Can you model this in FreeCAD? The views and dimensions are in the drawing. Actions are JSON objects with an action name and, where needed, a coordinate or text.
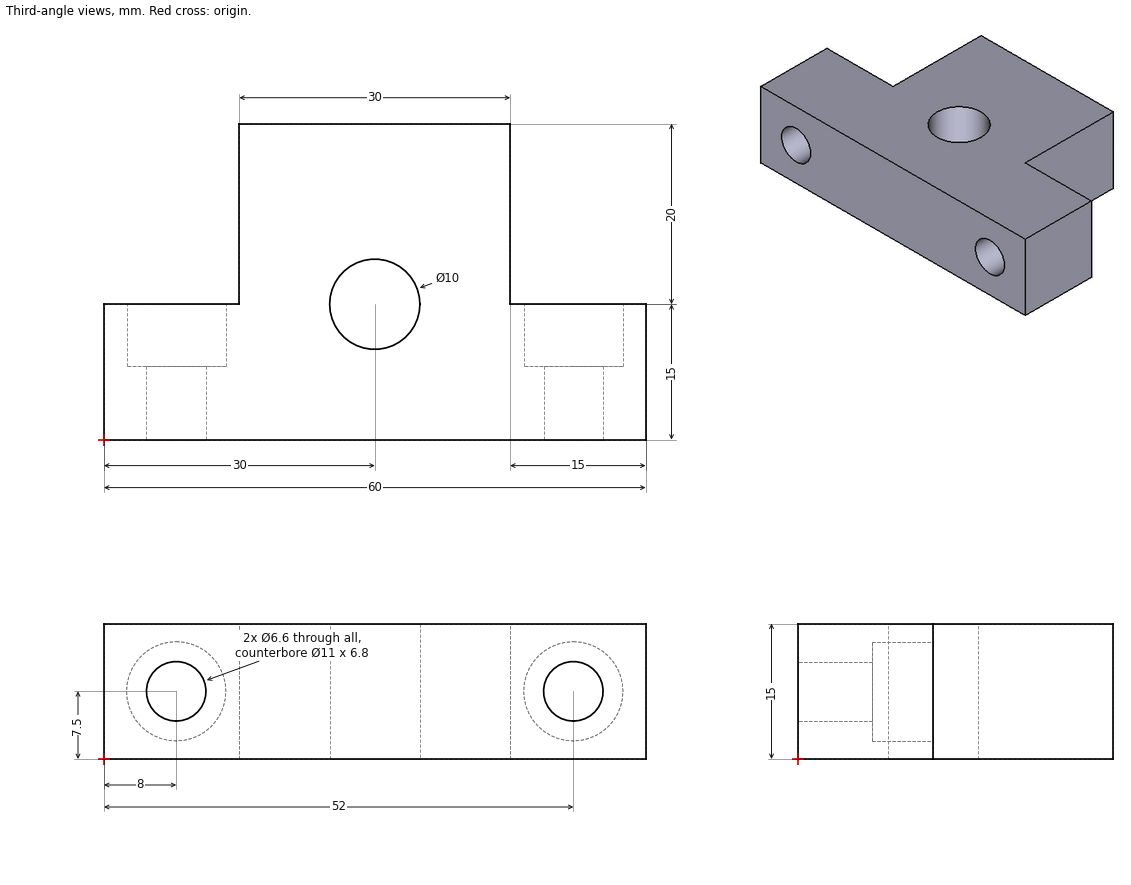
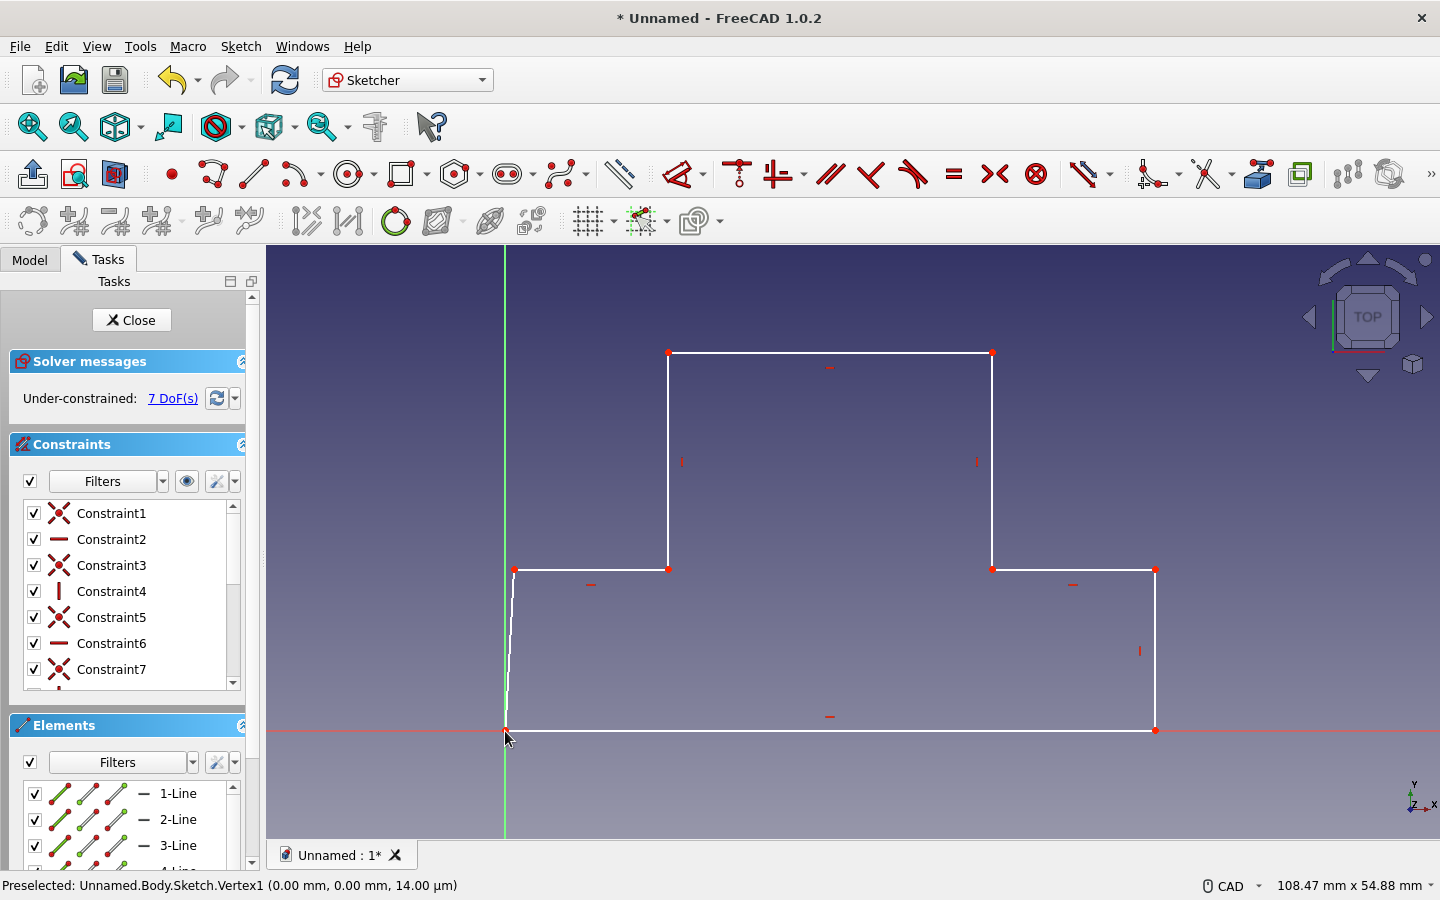
{"action": "left_click", "coordinate": [508, 683]}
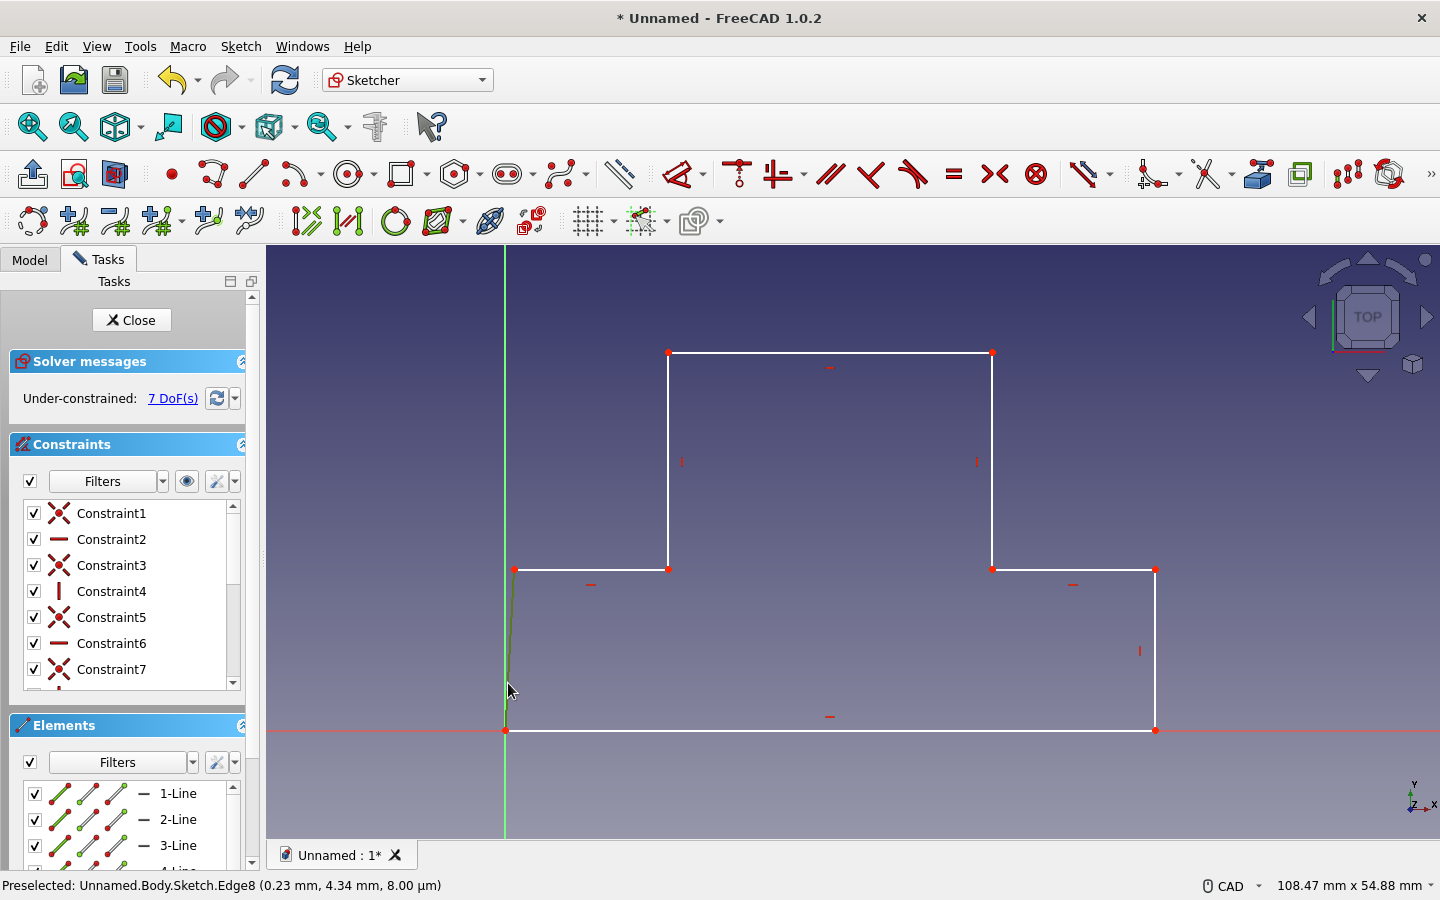
{"action": "key", "text": "v"}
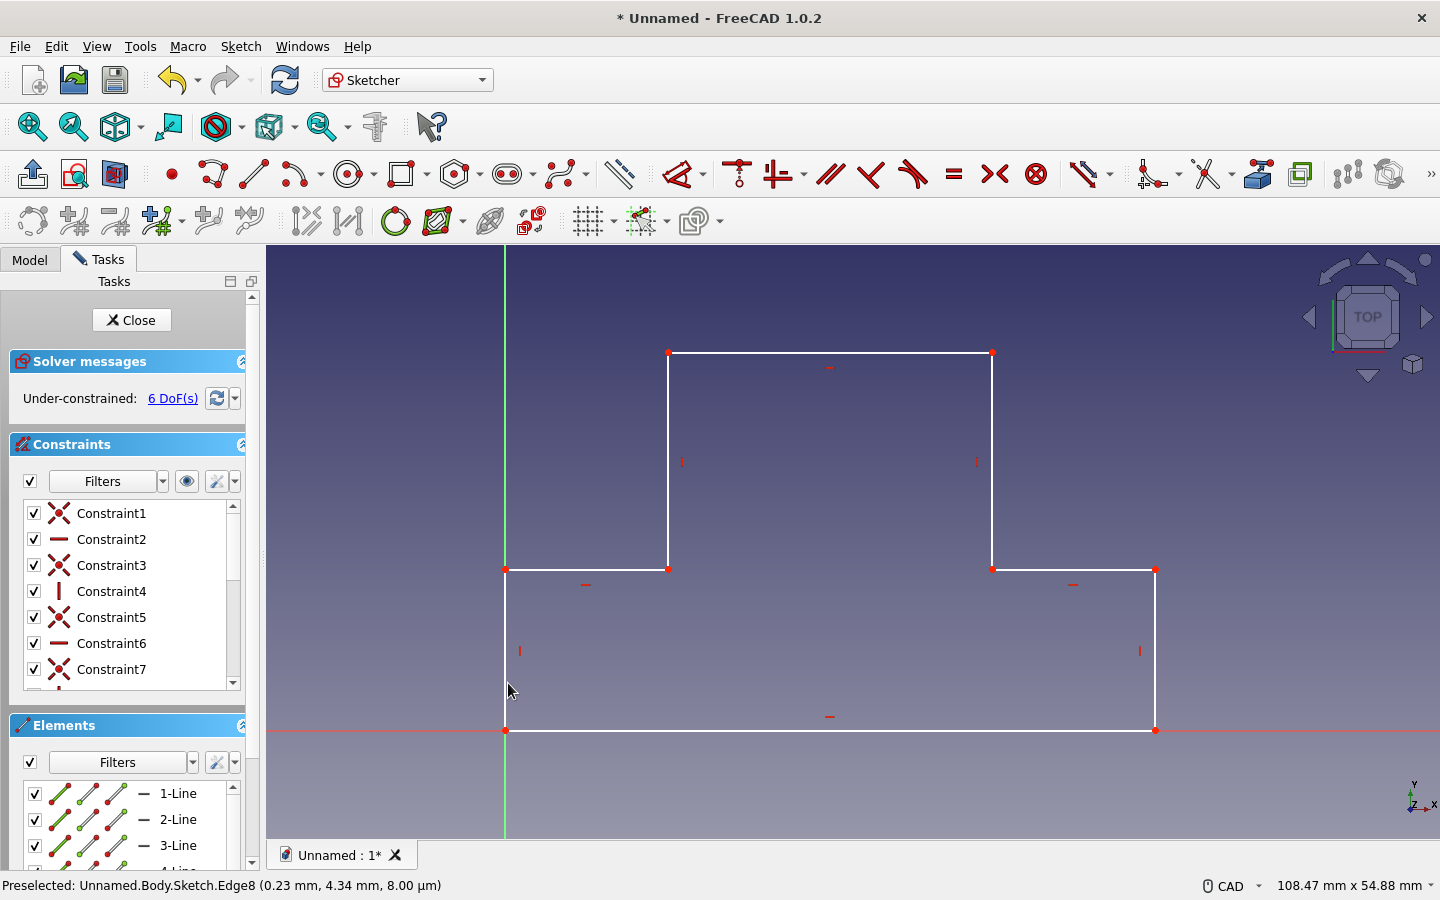
{"action": "left_click", "coordinate": [676, 174]}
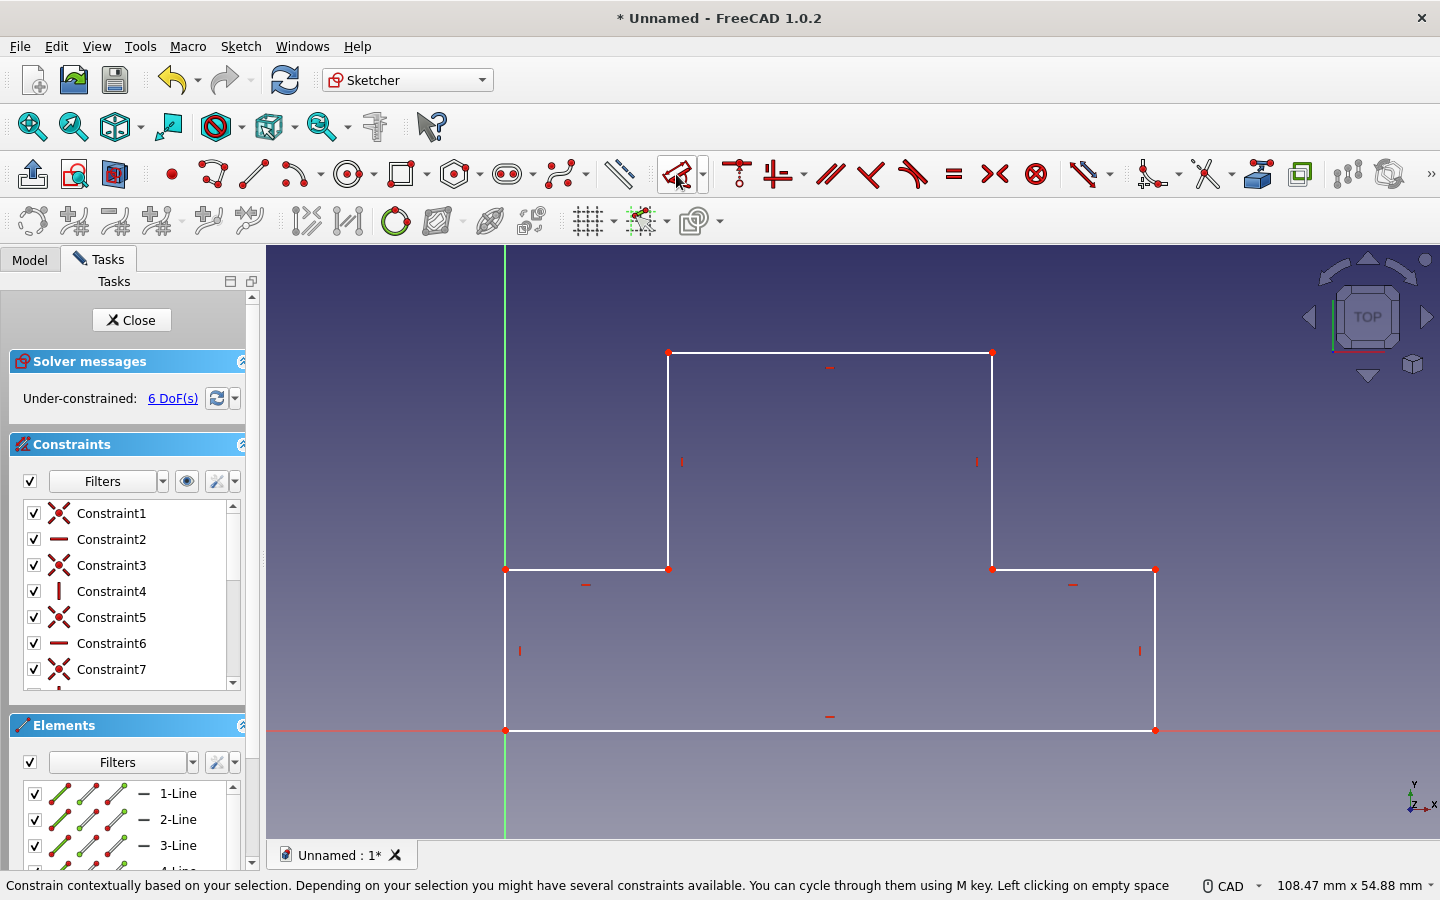
{"action": "left_click", "coordinate": [700, 731]}
{"action": "left_click", "coordinate": [830, 765]}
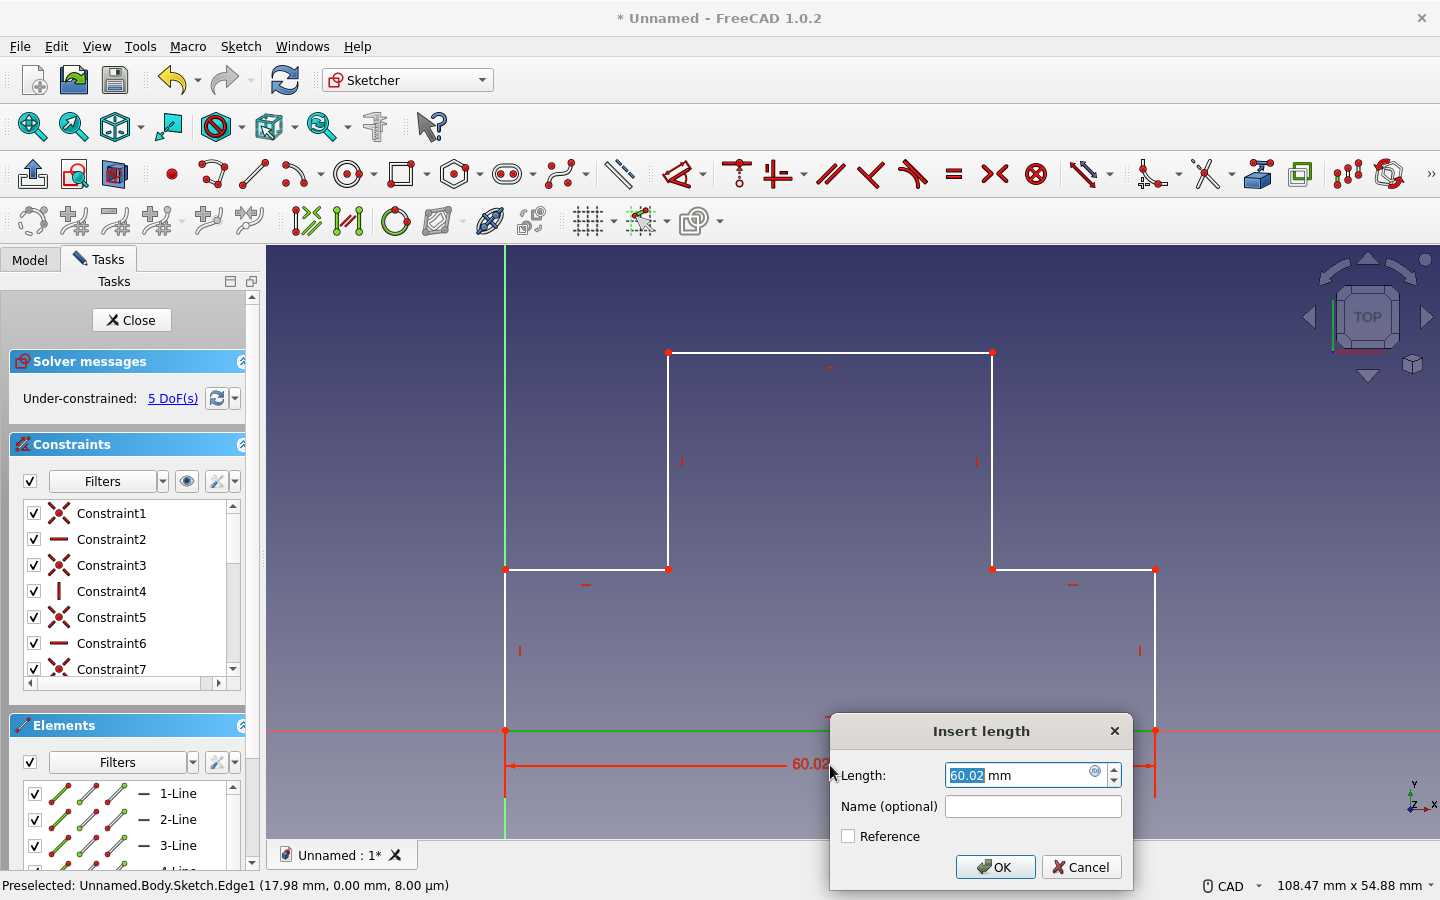
{"action": "type", "text": "60"}
{"action": "key", "text": "Return"}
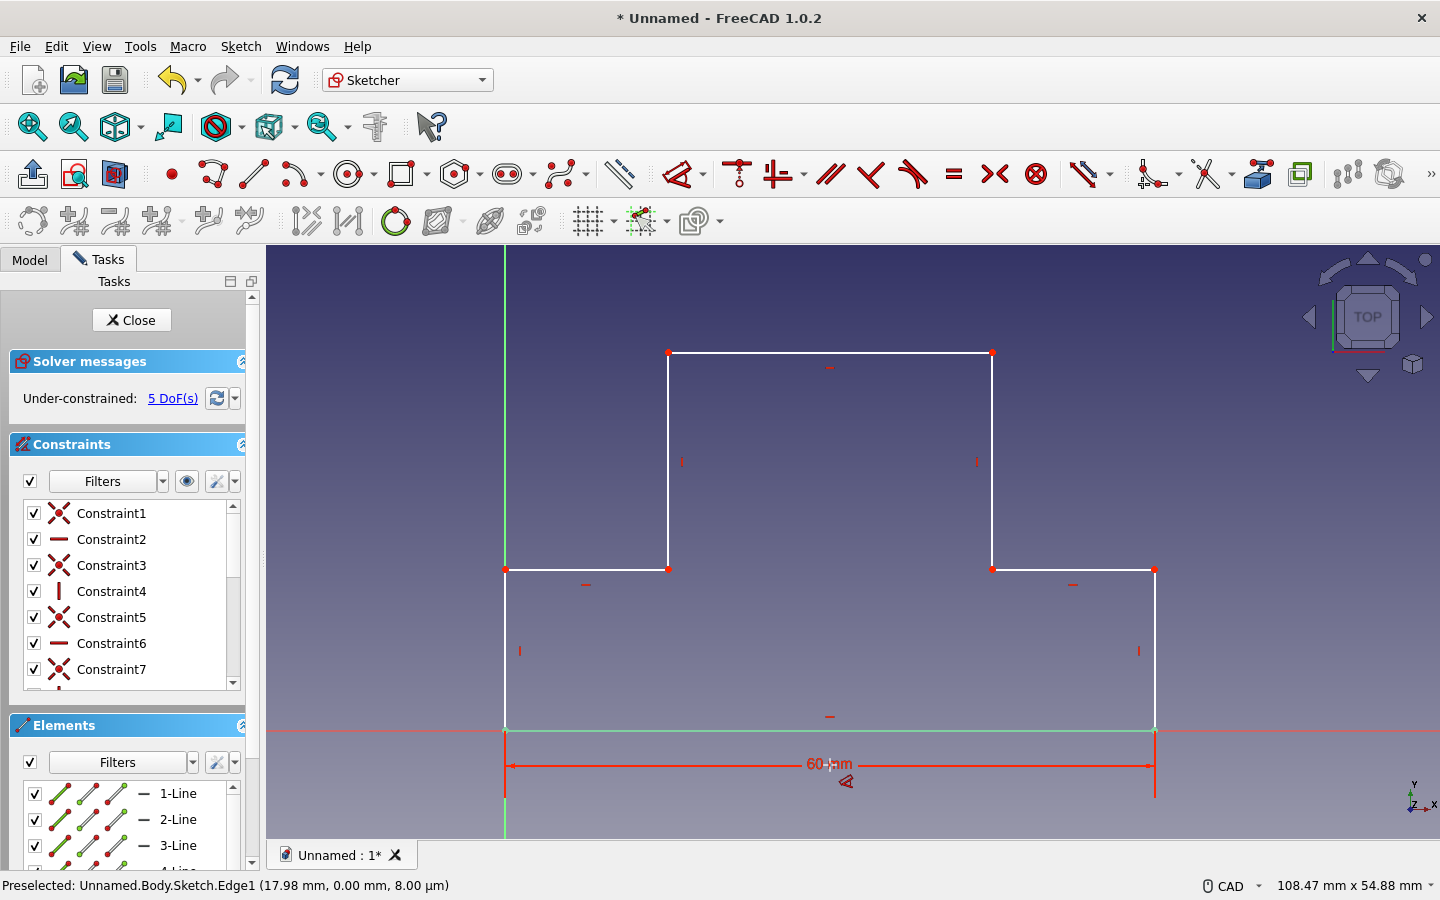
{"action": "left_click", "coordinate": [1155, 683]}
{"action": "left_click", "coordinate": [1189, 650]}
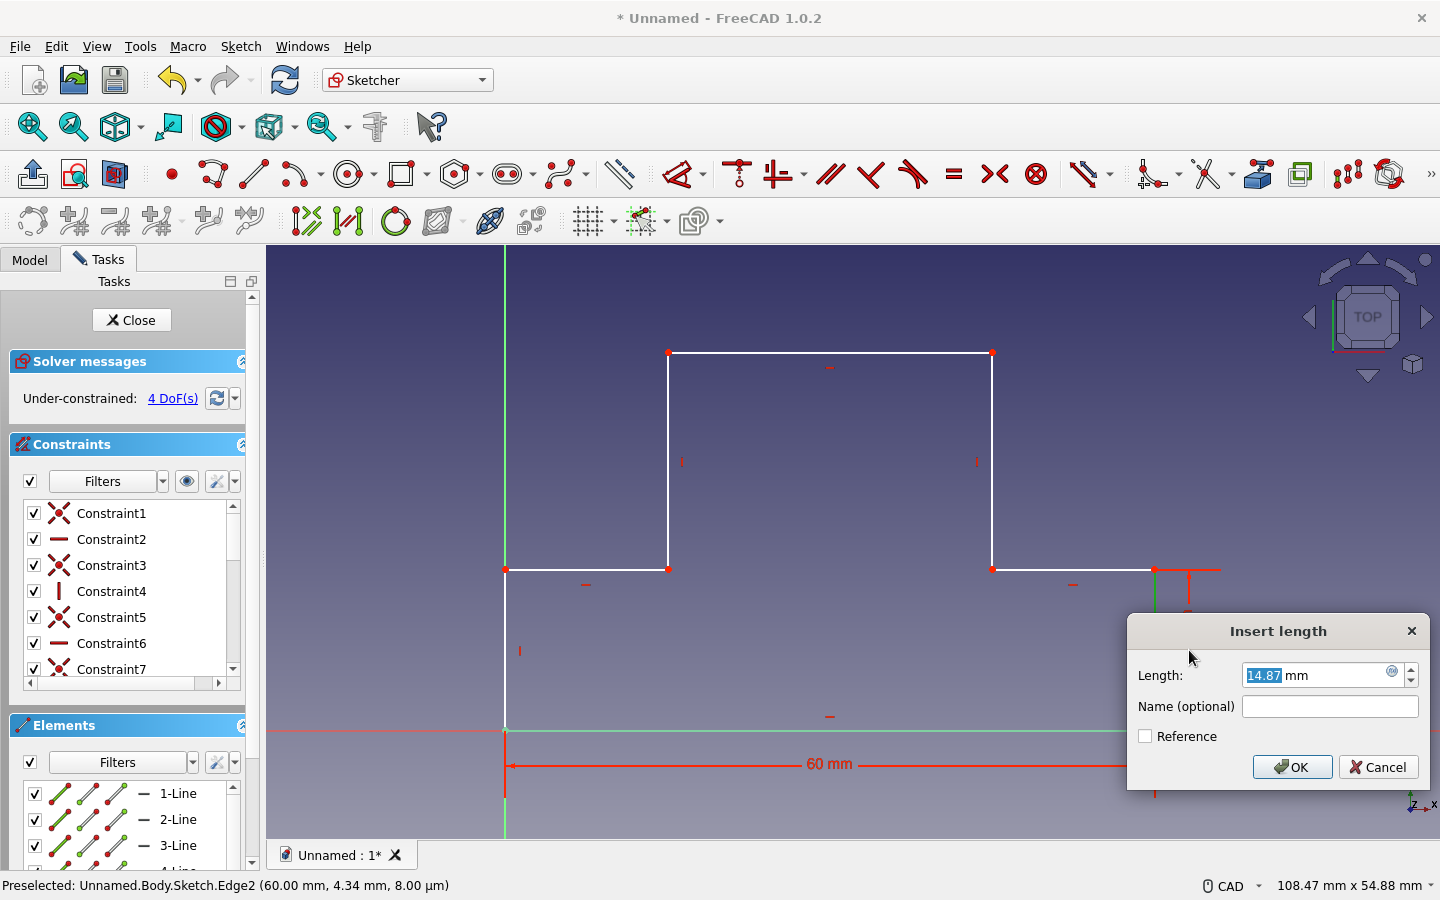
{"action": "type", "text": "15"}
{"action": "key", "text": "Return"}